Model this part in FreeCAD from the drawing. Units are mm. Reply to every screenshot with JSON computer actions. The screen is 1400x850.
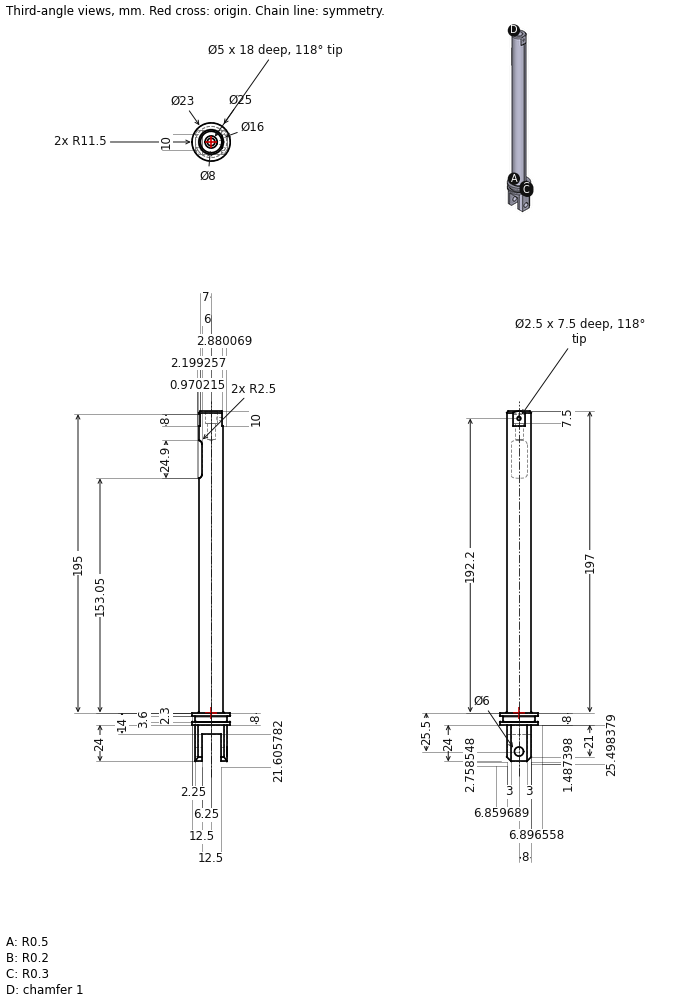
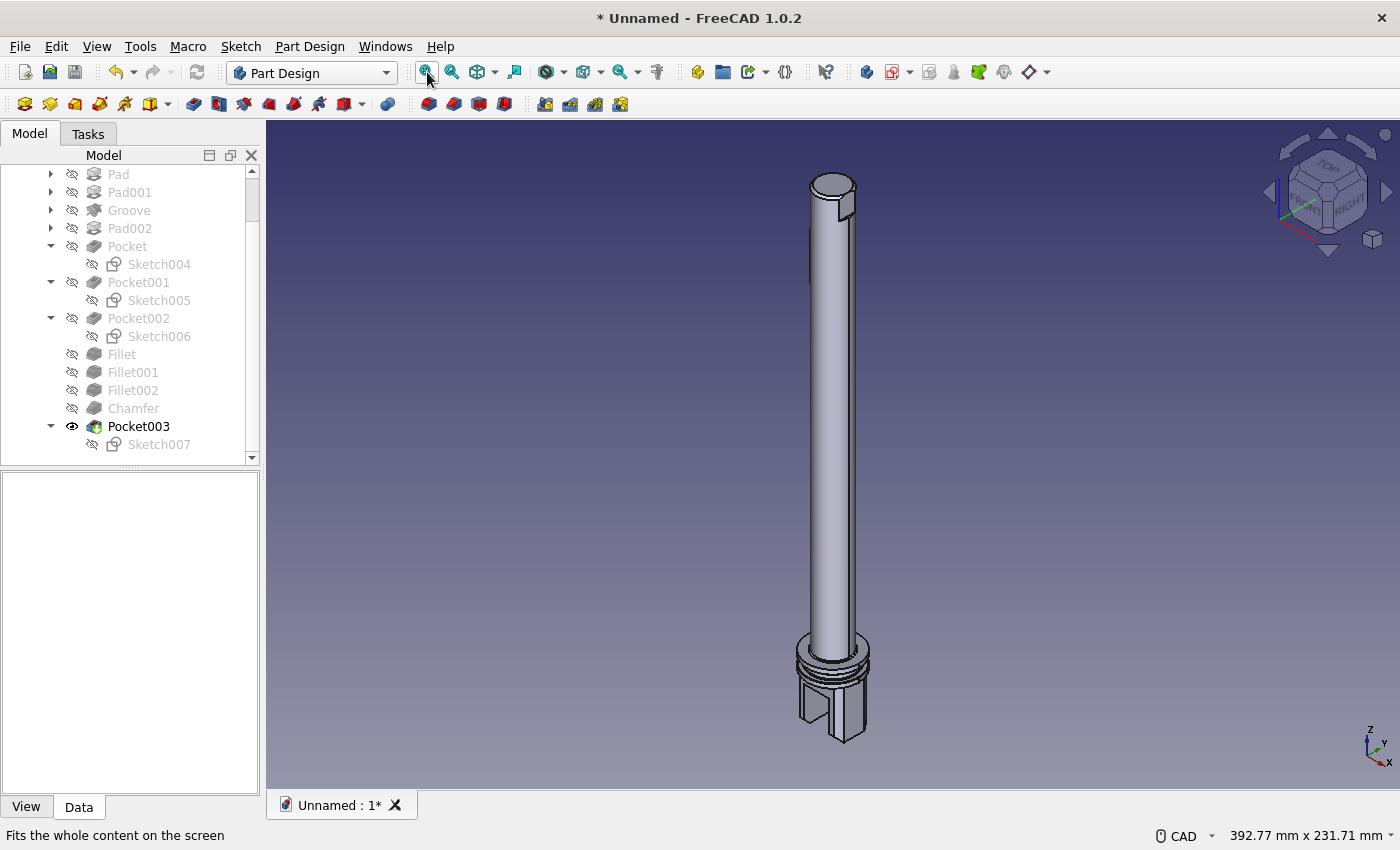
{"action": "left_click", "coordinate": [854, 699]}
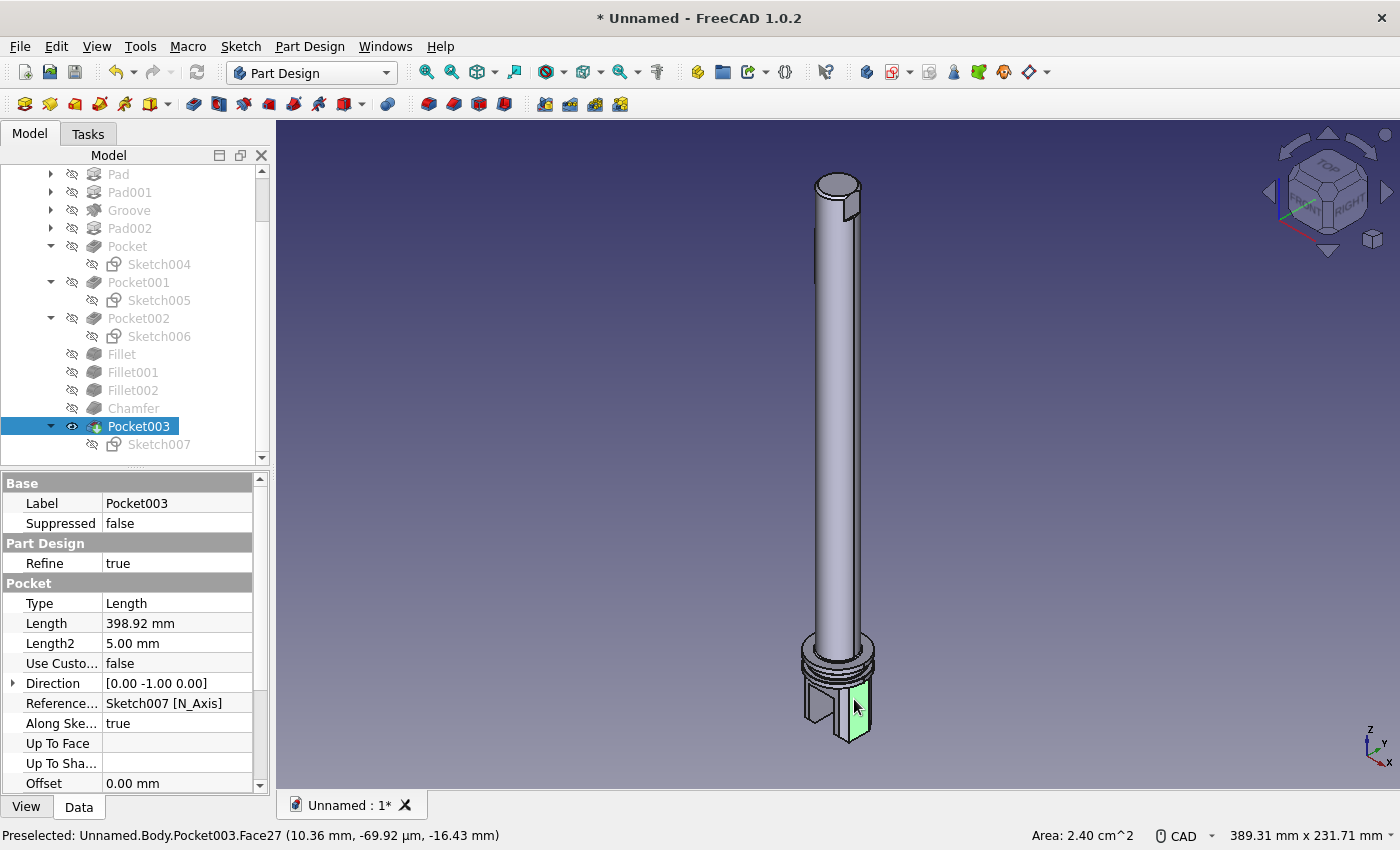
{"action": "left_click", "coordinate": [892, 72]}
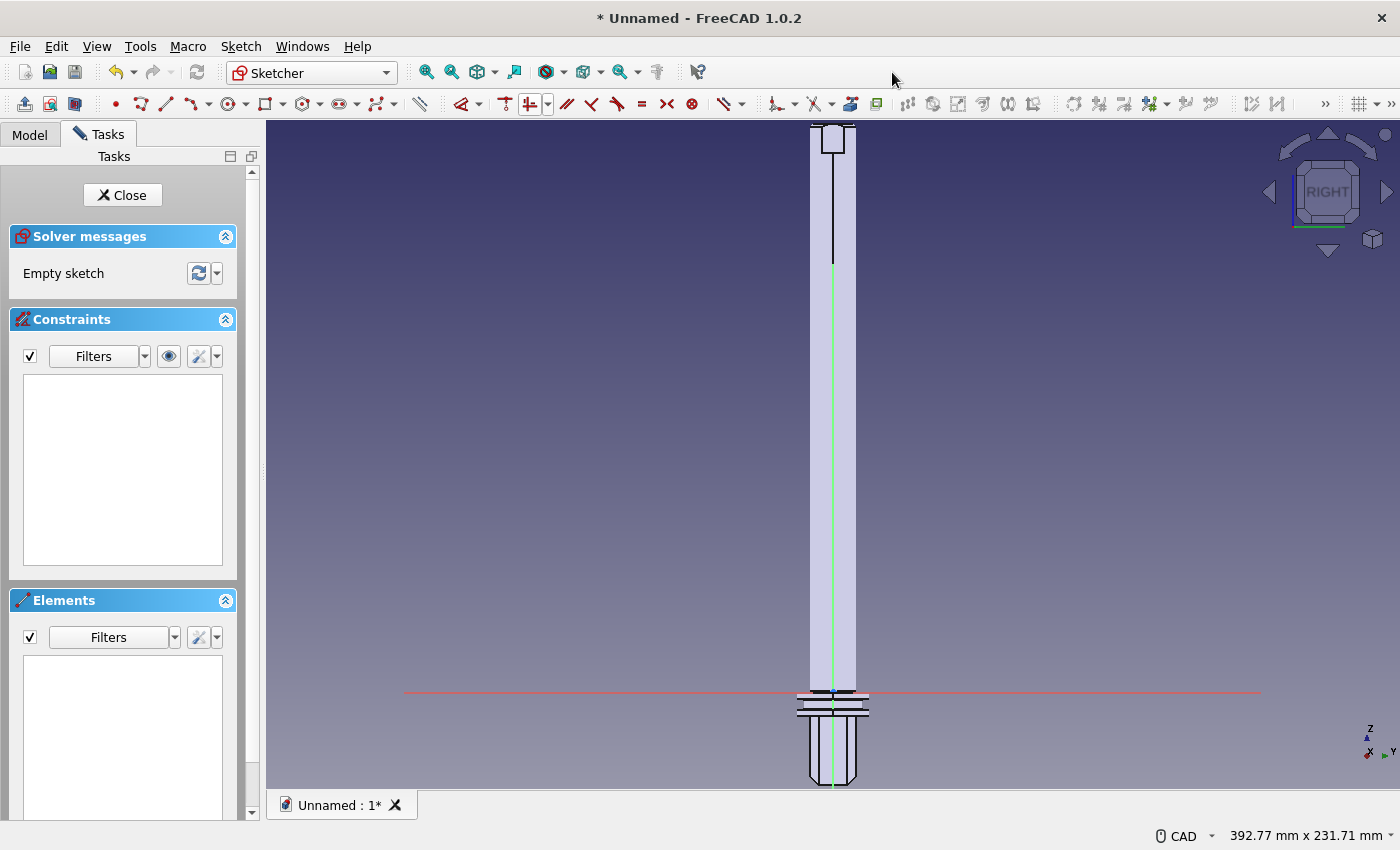
{"action": "left_click", "coordinate": [75, 104]}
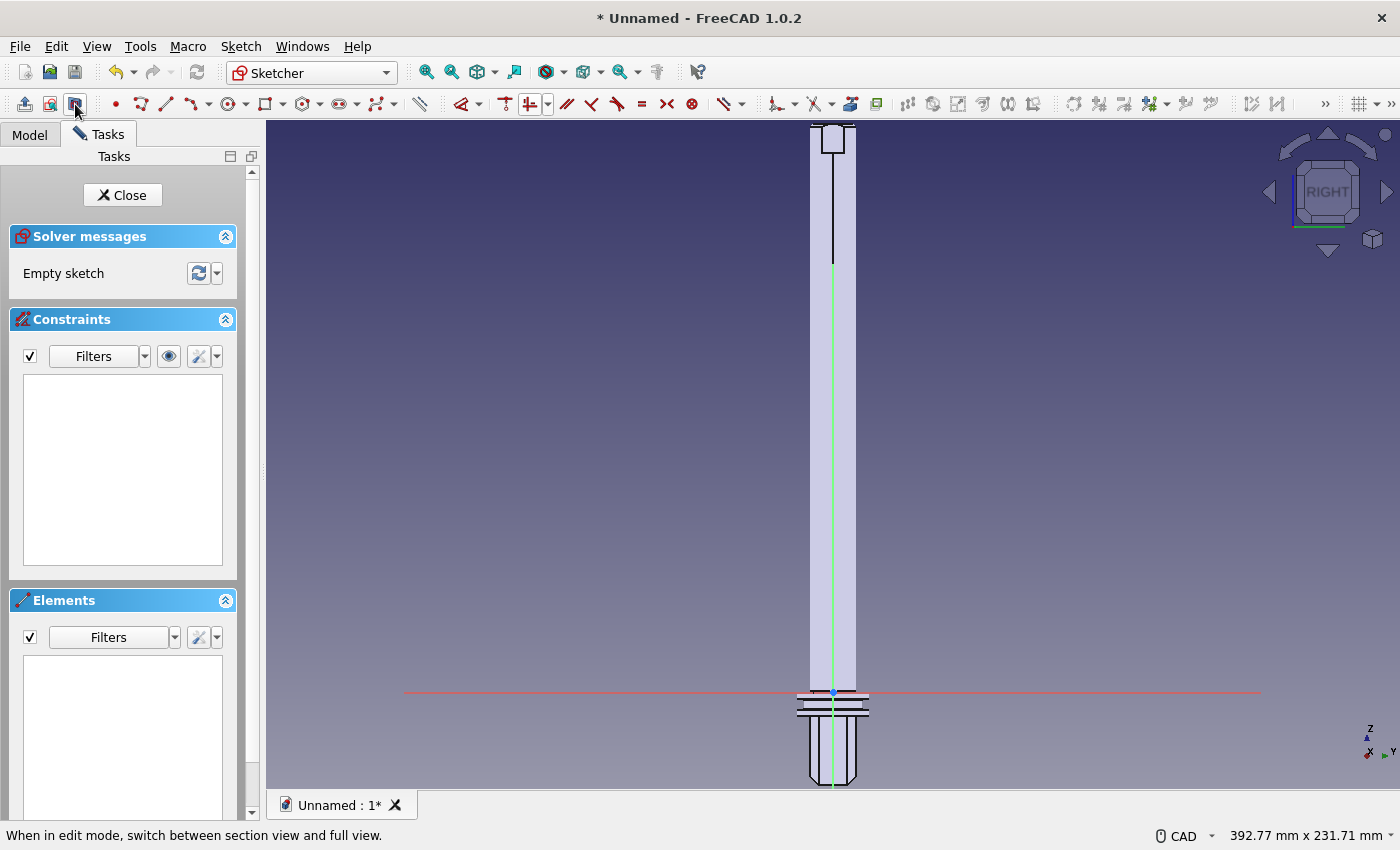
{"action": "scroll", "coordinate": [764, 454], "scroll_direction": "down", "scroll_amount": 5}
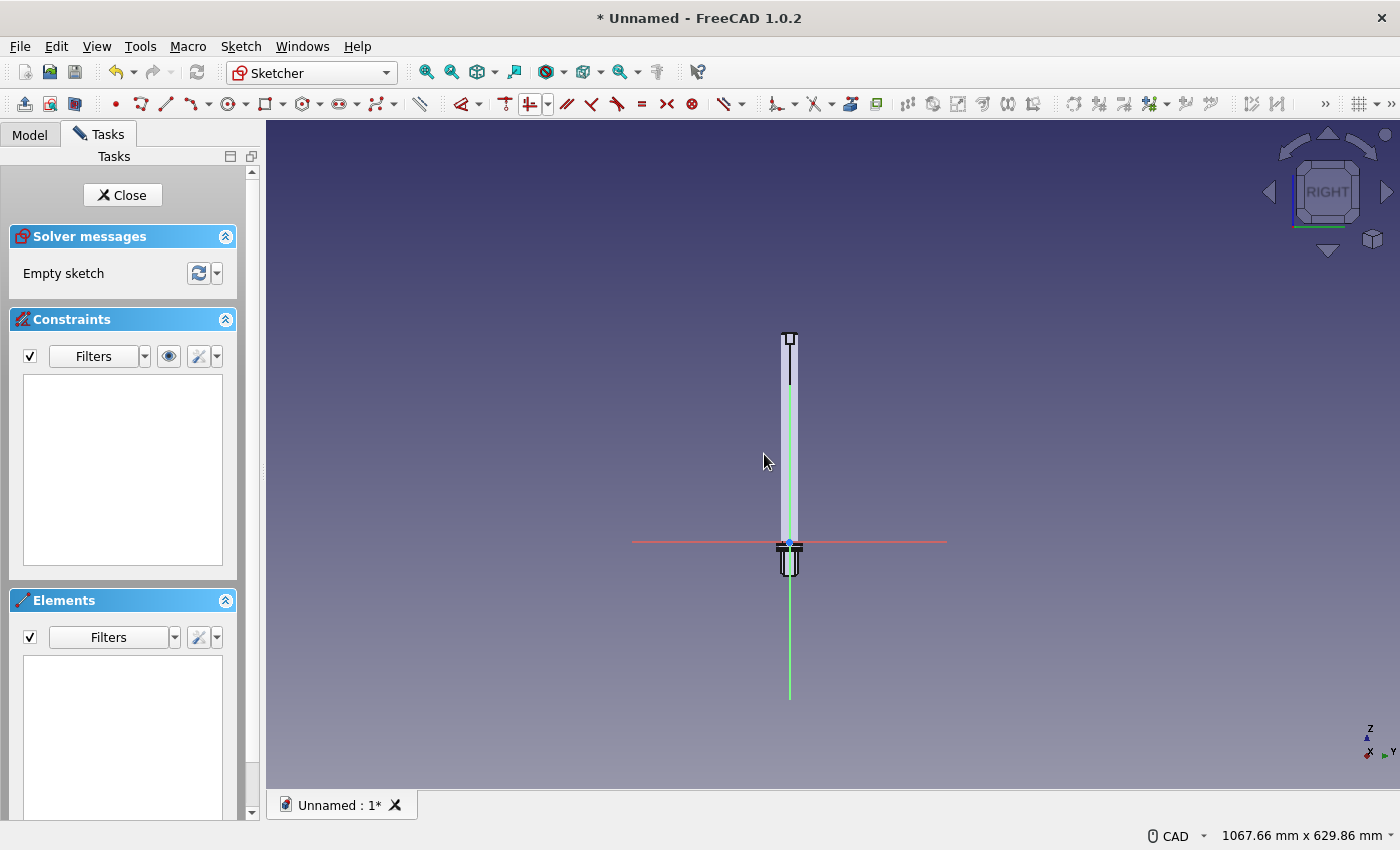
{"action": "scroll", "coordinate": [791, 575], "scroll_direction": "up", "scroll_amount": 15}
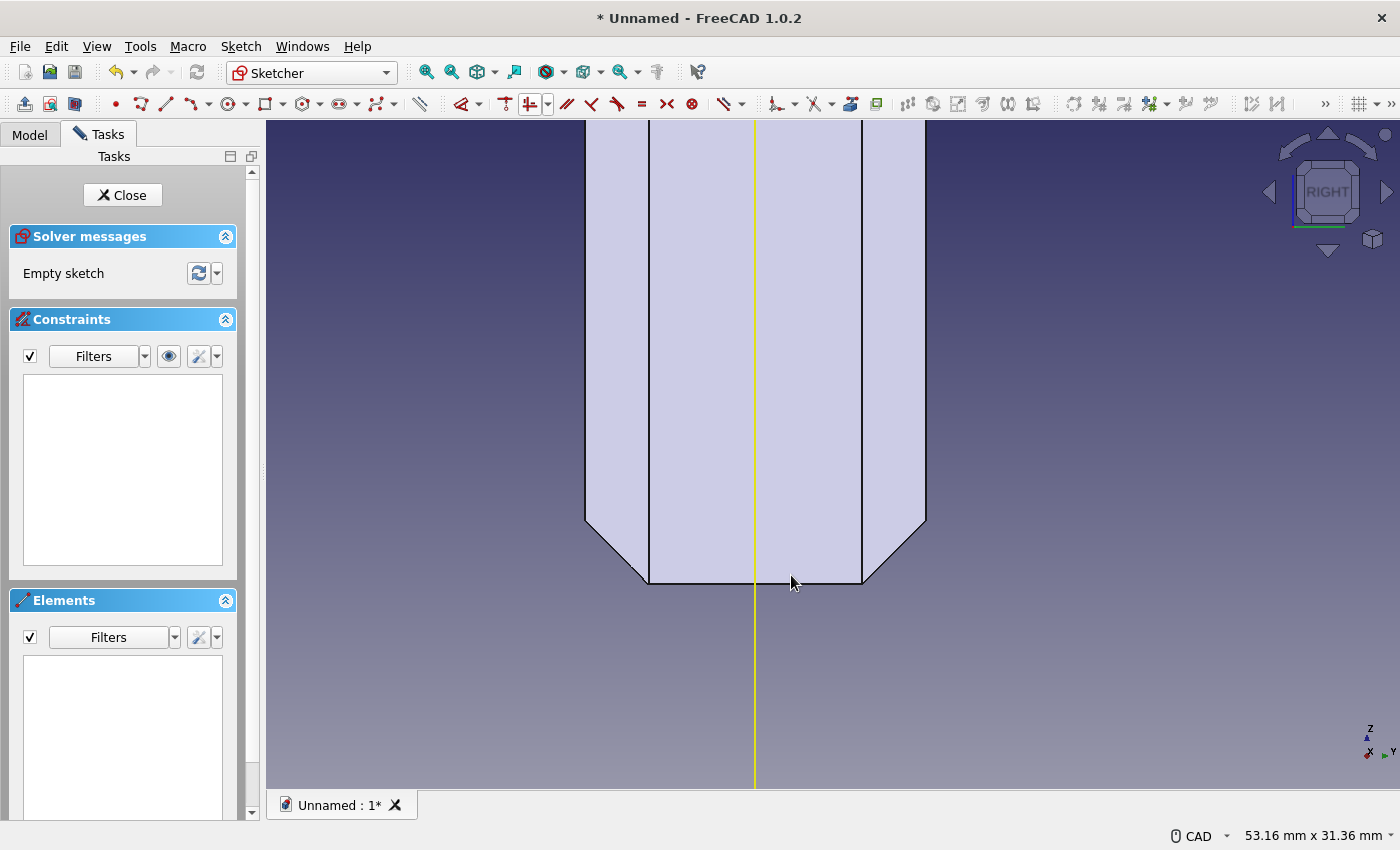
{"action": "scroll", "coordinate": [751, 442], "scroll_direction": "up", "scroll_amount": 6}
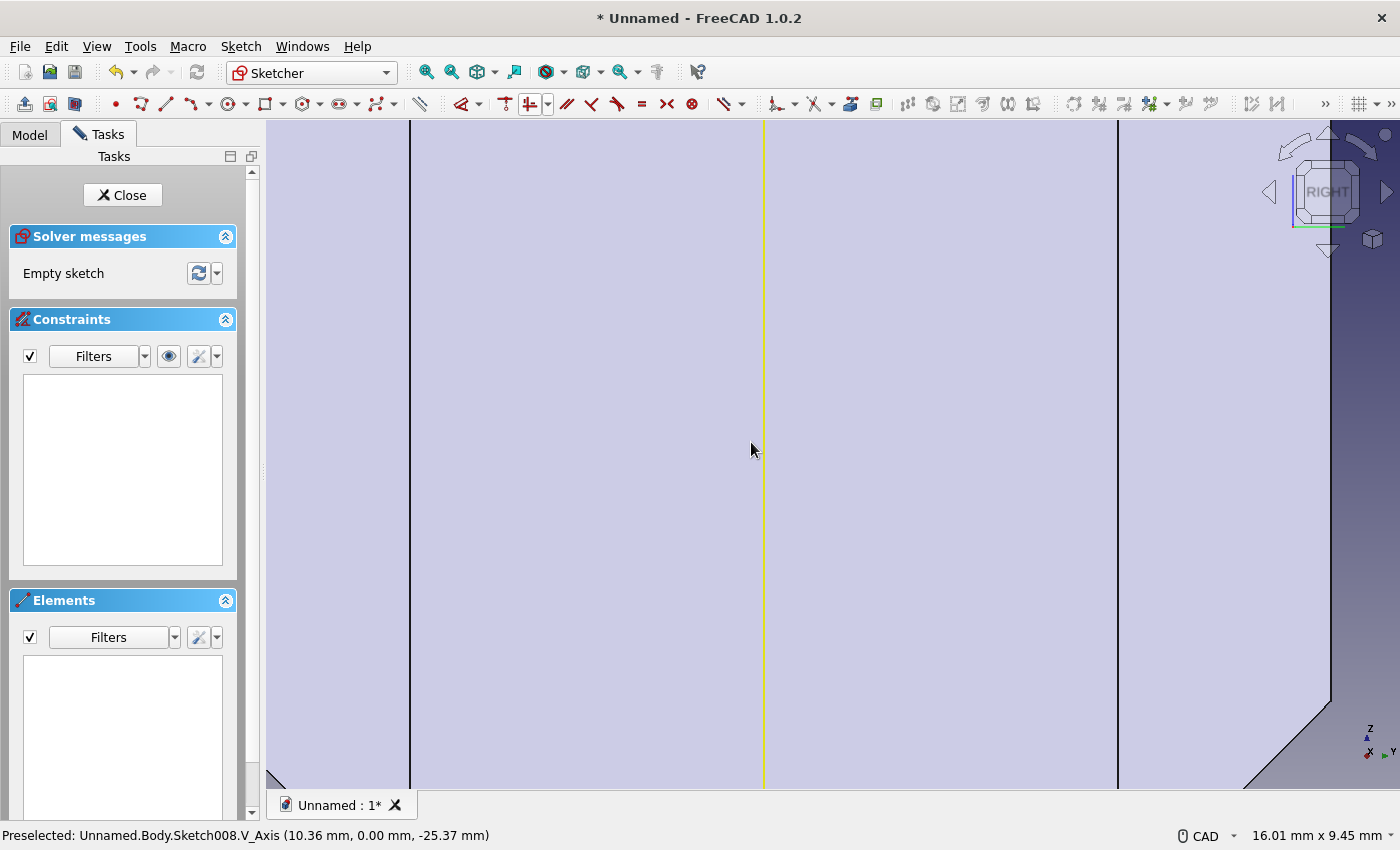
{"action": "left_click", "coordinate": [228, 104]}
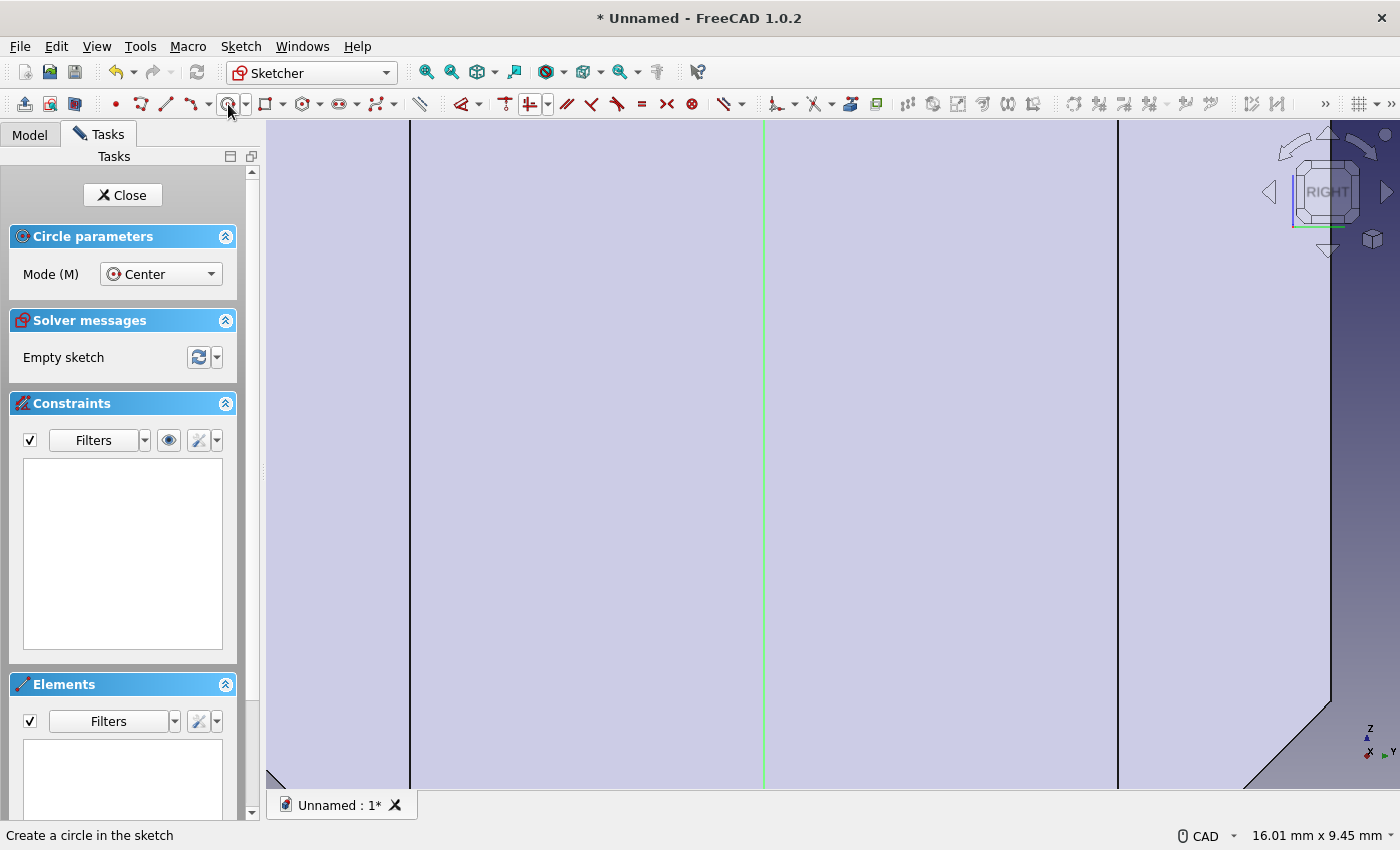
{"action": "left_click", "coordinate": [764, 453]}
{"action": "mouse_move", "coordinate": [914, 303]}